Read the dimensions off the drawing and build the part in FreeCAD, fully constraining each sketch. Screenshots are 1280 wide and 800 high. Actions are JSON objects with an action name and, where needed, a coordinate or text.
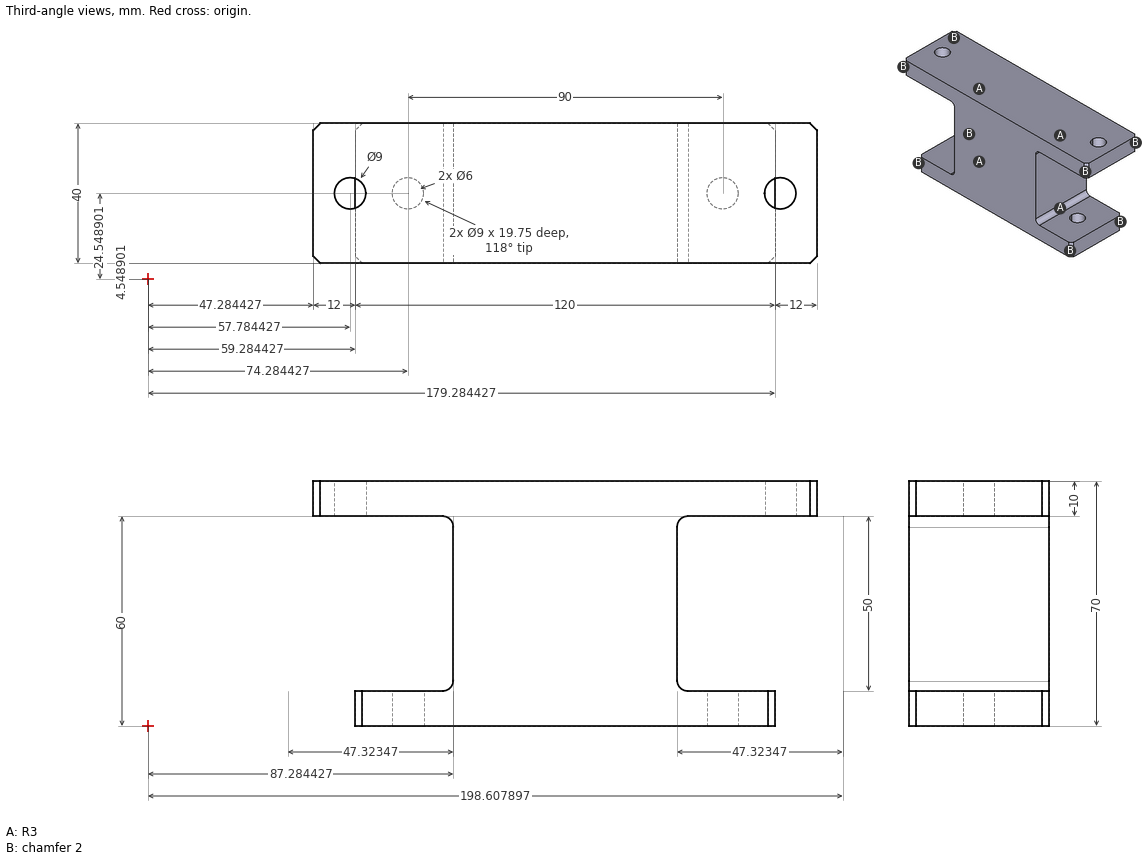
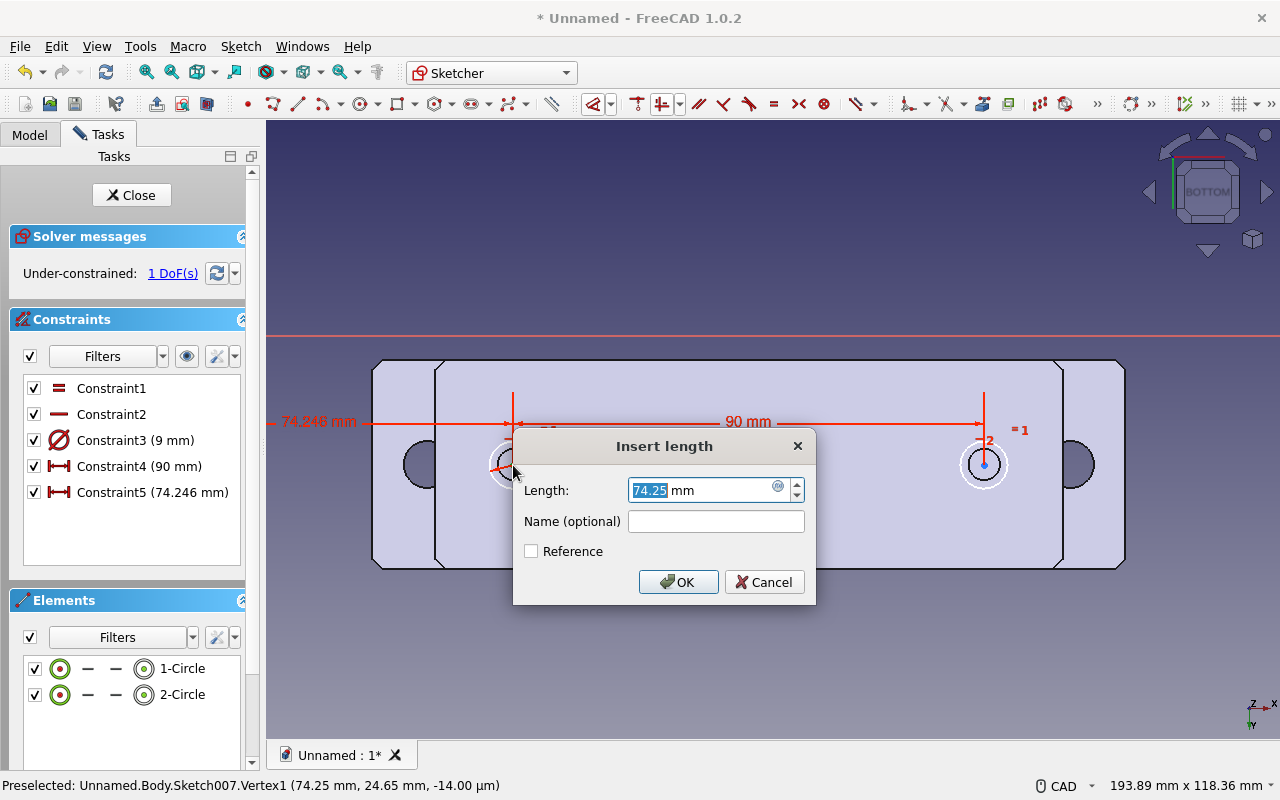
{"action": "type", "text": "74.284427"}
{"action": "key", "text": "Return"}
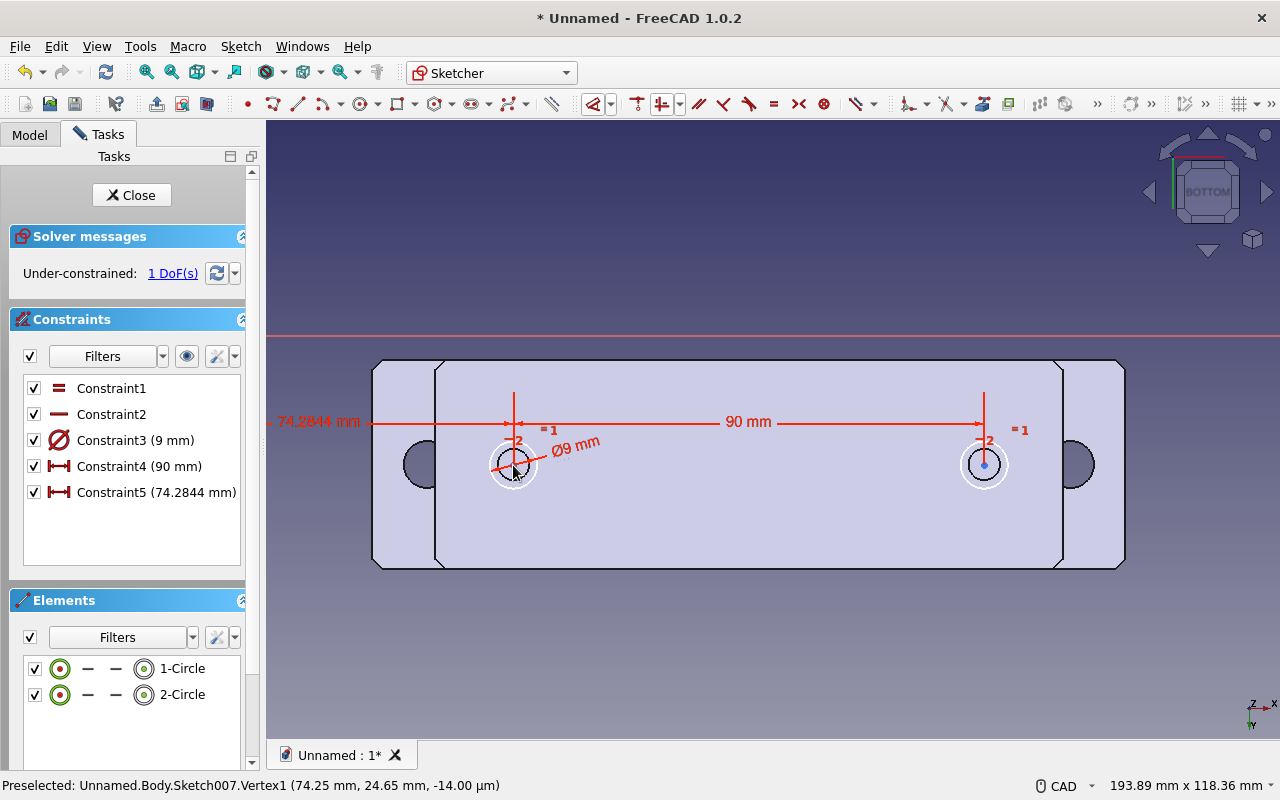
{"action": "left_click", "coordinate": [514, 465]}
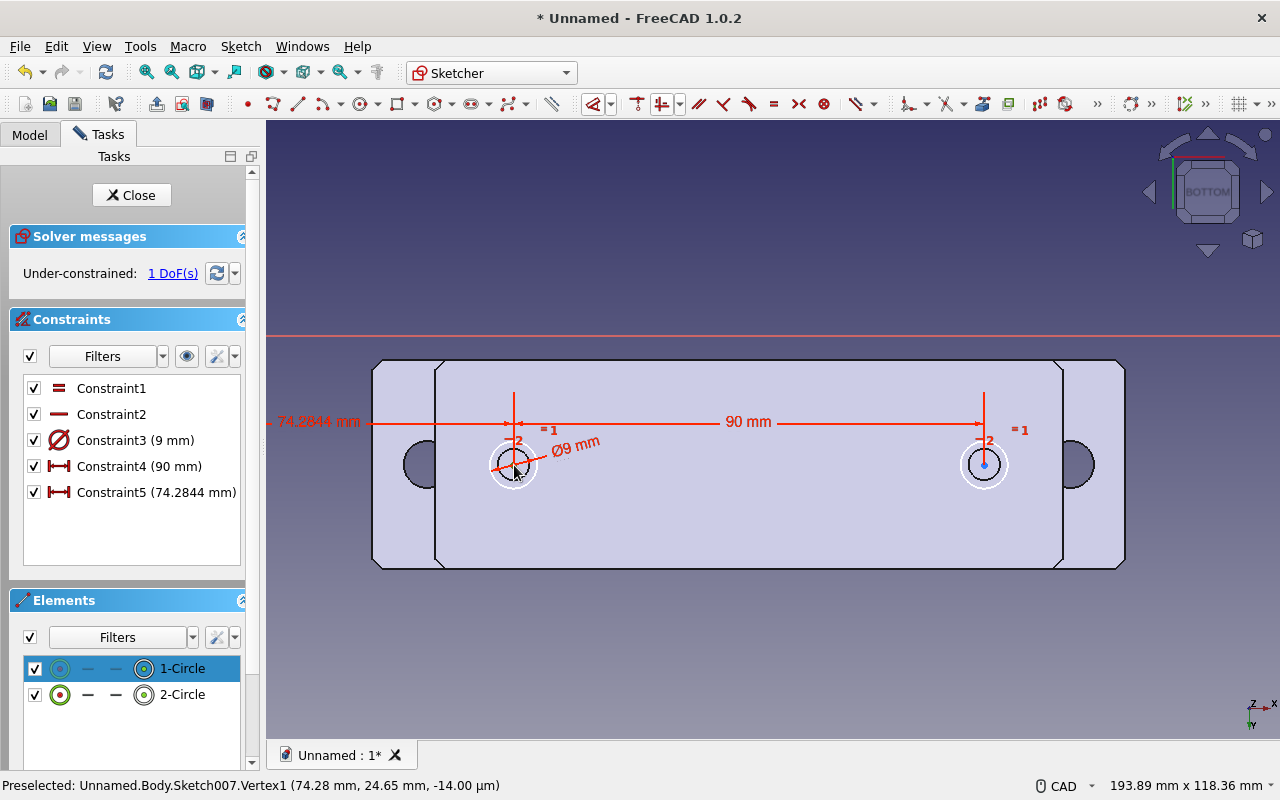
{"action": "key", "text": "i"}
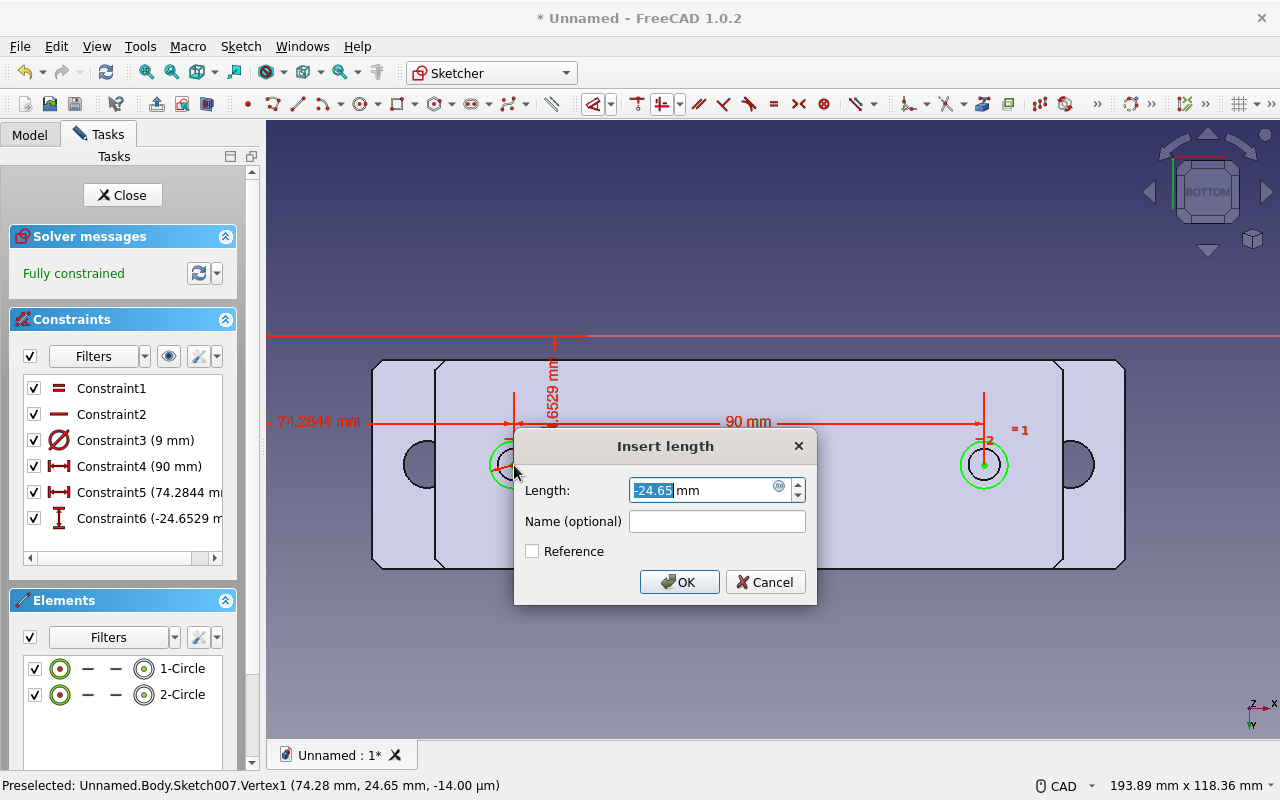
{"action": "type", "text": "-24.548901"}
{"action": "key", "text": "Return"}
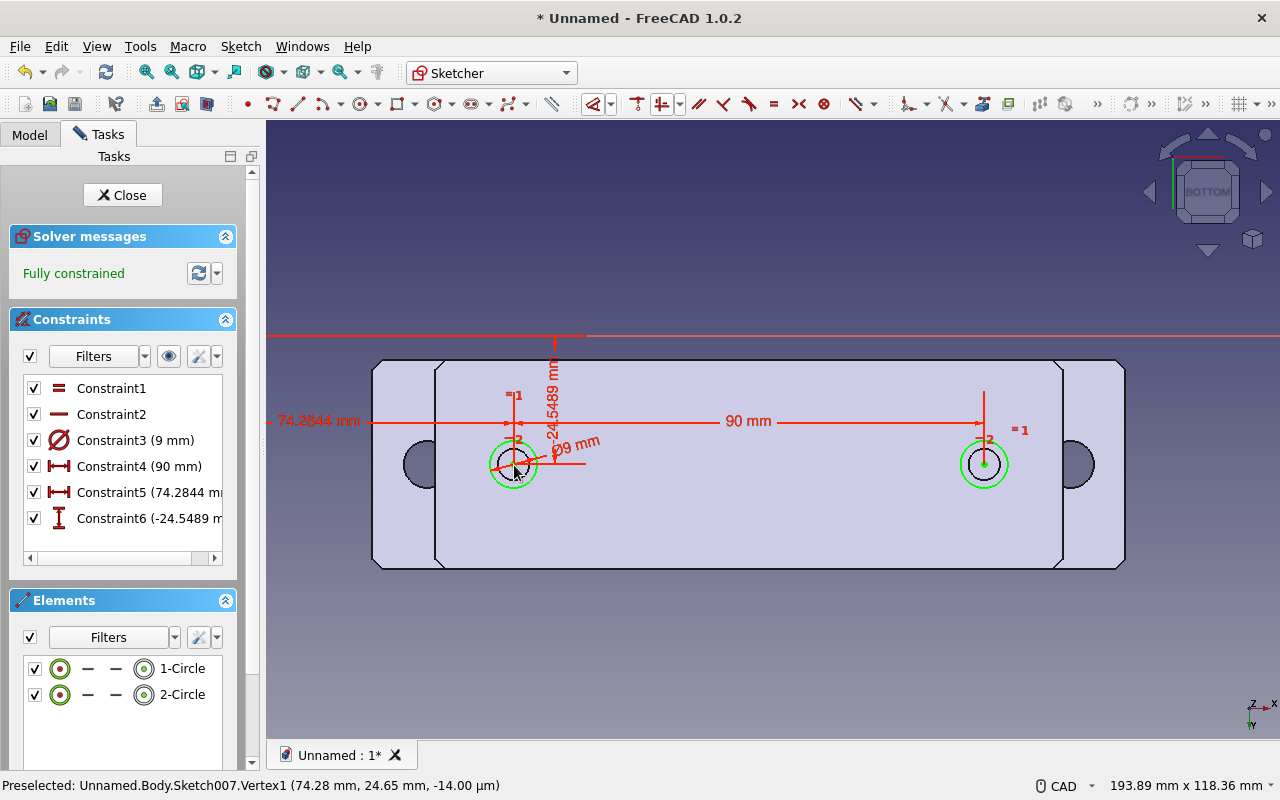
{"action": "left_click", "coordinate": [123, 195]}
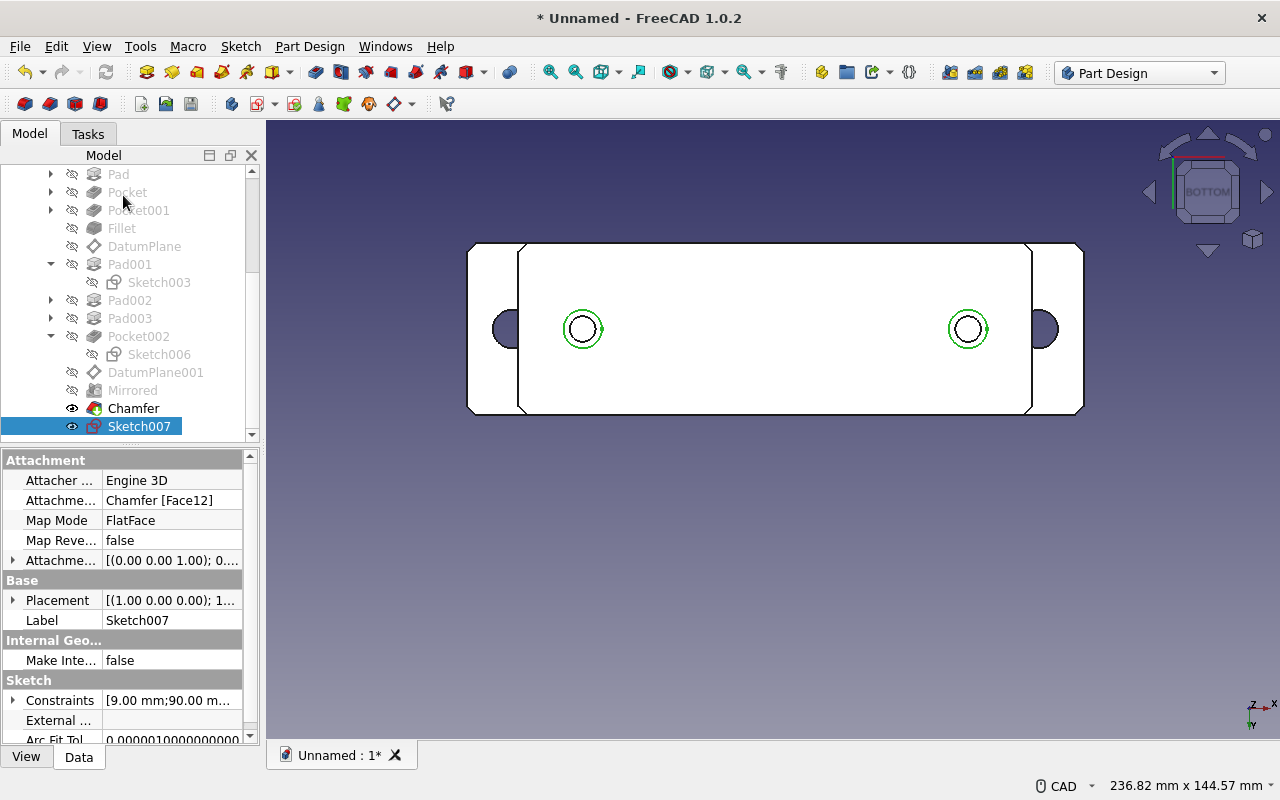
{"action": "left_click", "coordinate": [341, 72]}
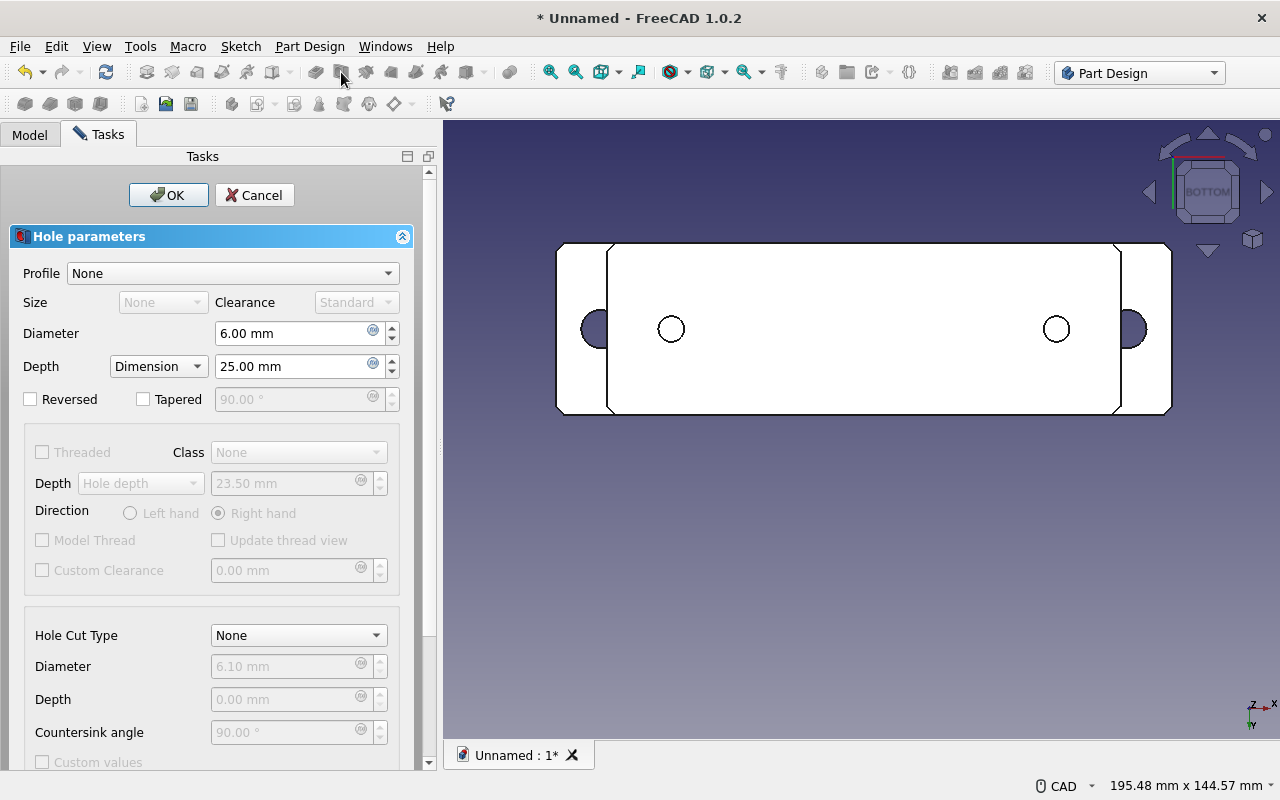
{"action": "triple_click", "coordinate": [300, 334]}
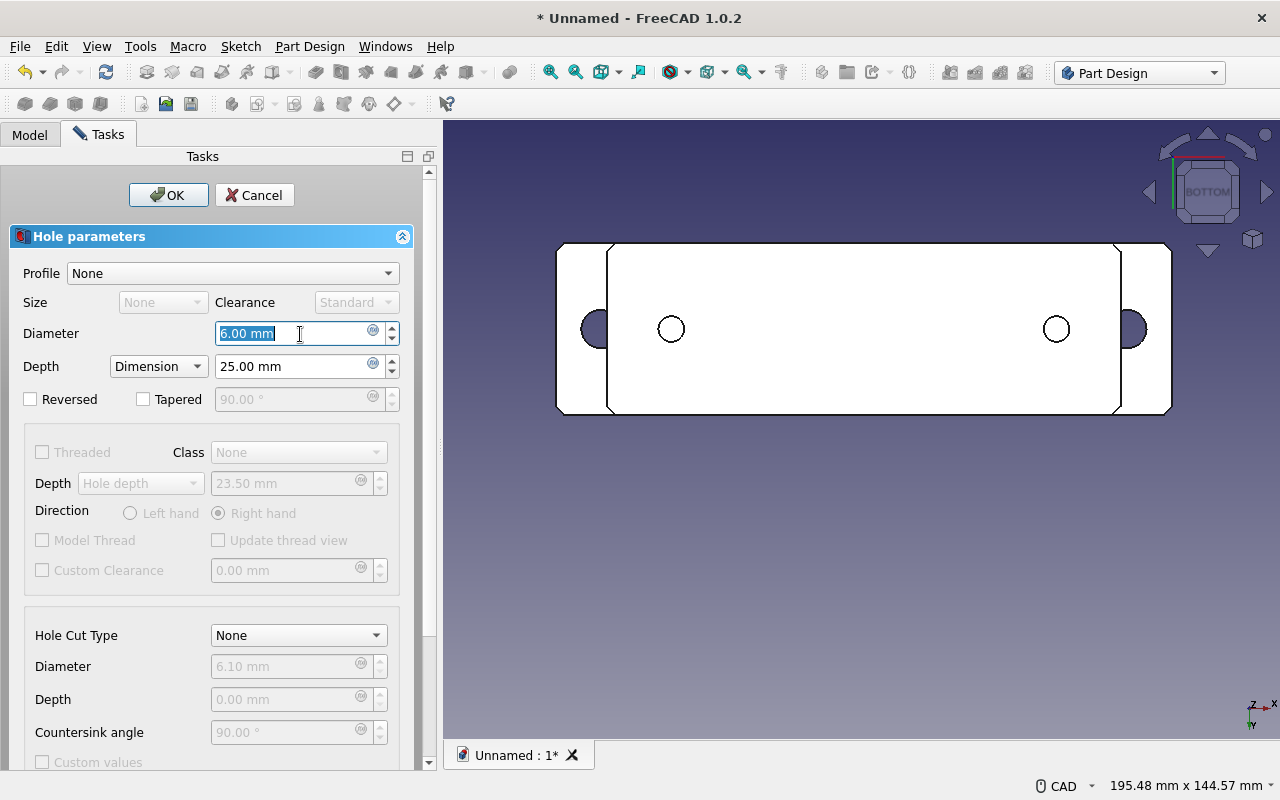
{"action": "type", "text": "9"}
{"action": "key", "text": "Tab"}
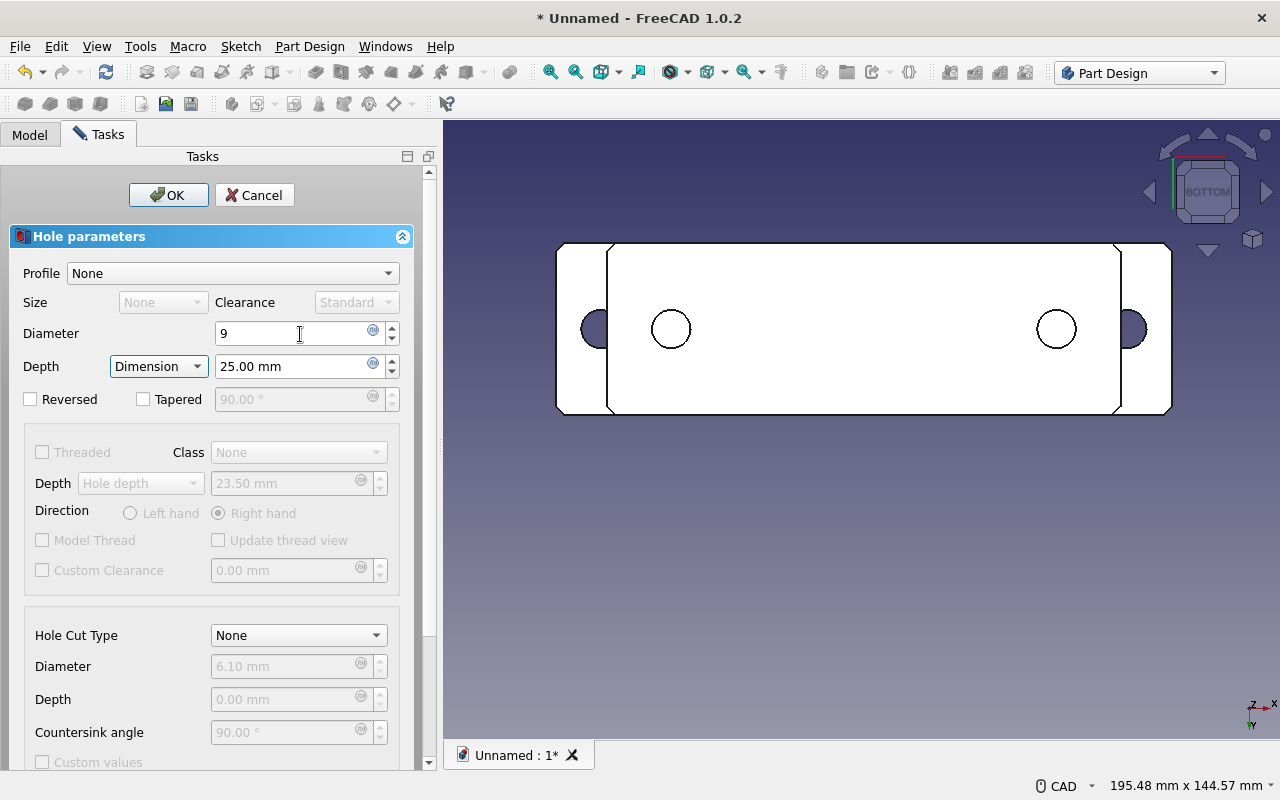
{"action": "triple_click", "coordinate": [300, 366]}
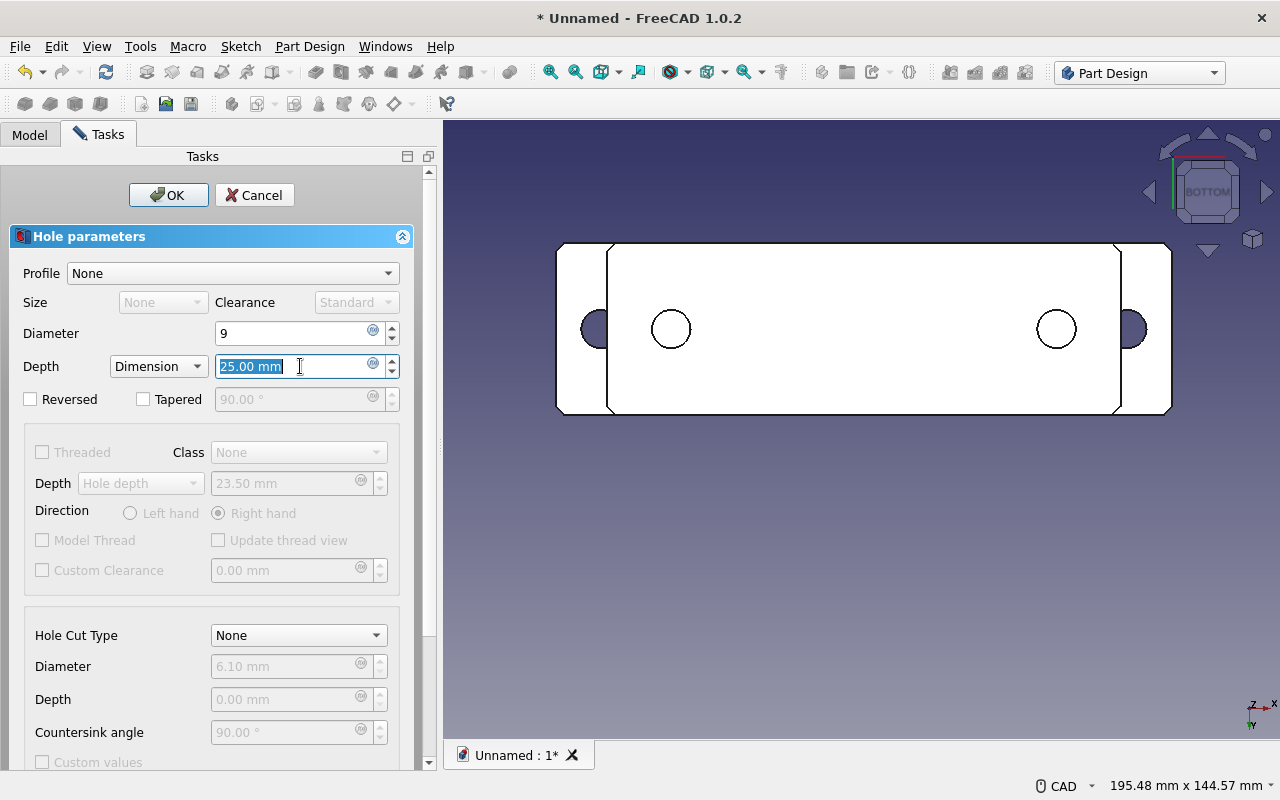
{"action": "type", "text": "19.75"}
{"action": "key", "text": "Tab"}